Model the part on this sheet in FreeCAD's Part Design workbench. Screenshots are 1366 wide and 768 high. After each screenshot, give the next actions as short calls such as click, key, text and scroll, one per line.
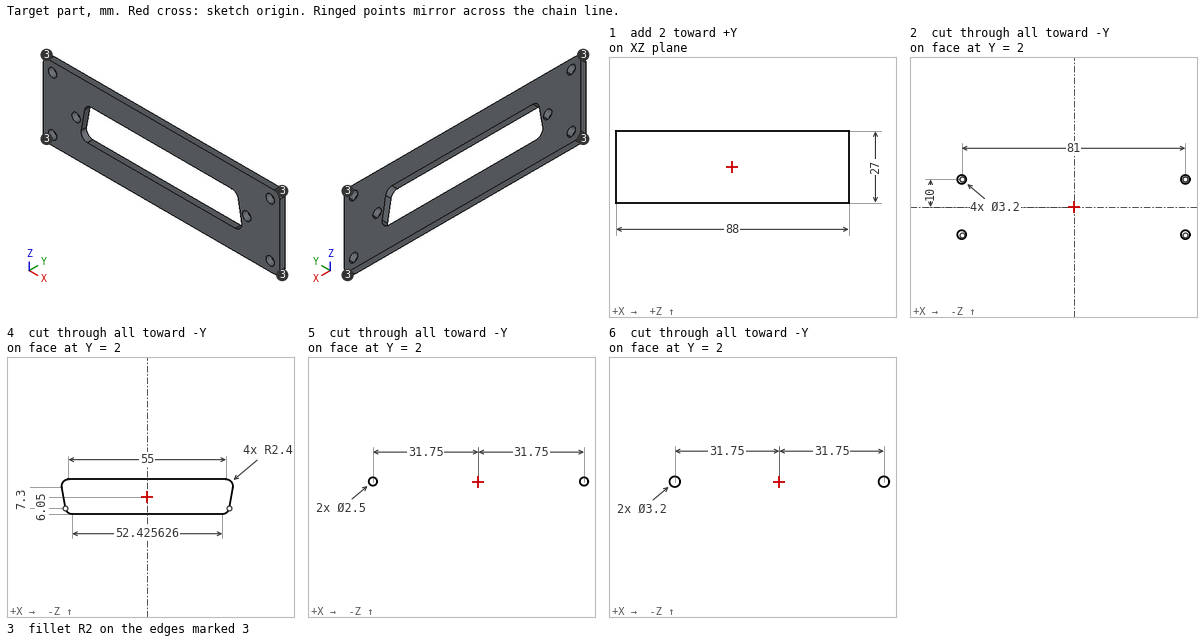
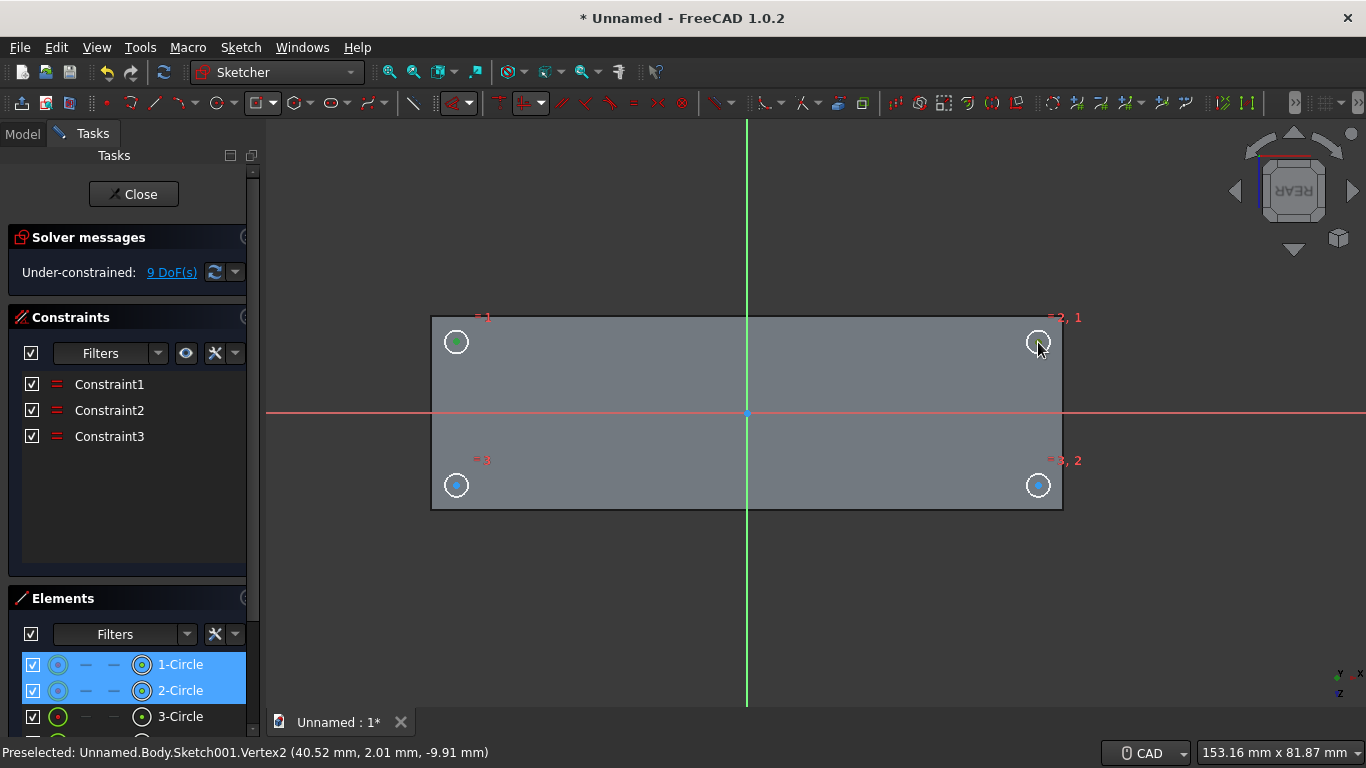
click(747, 641)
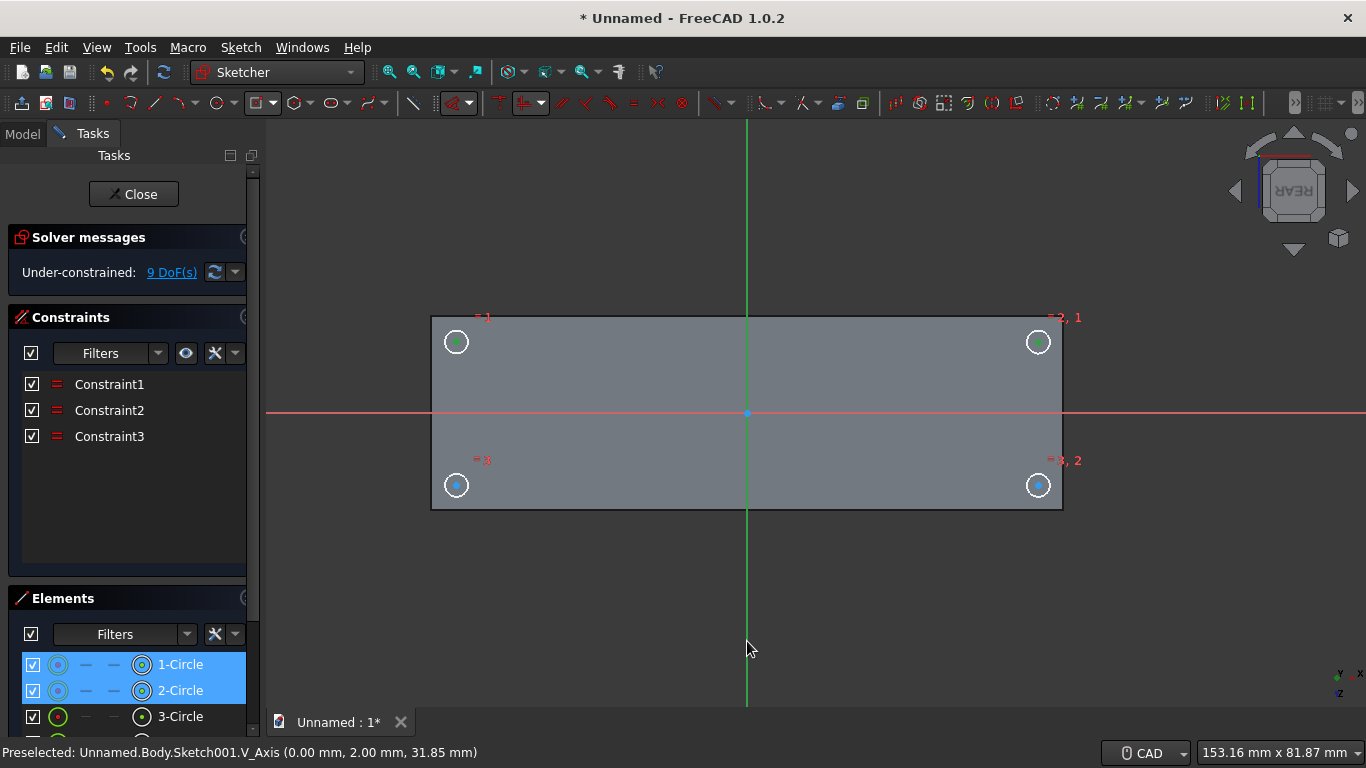
key(s)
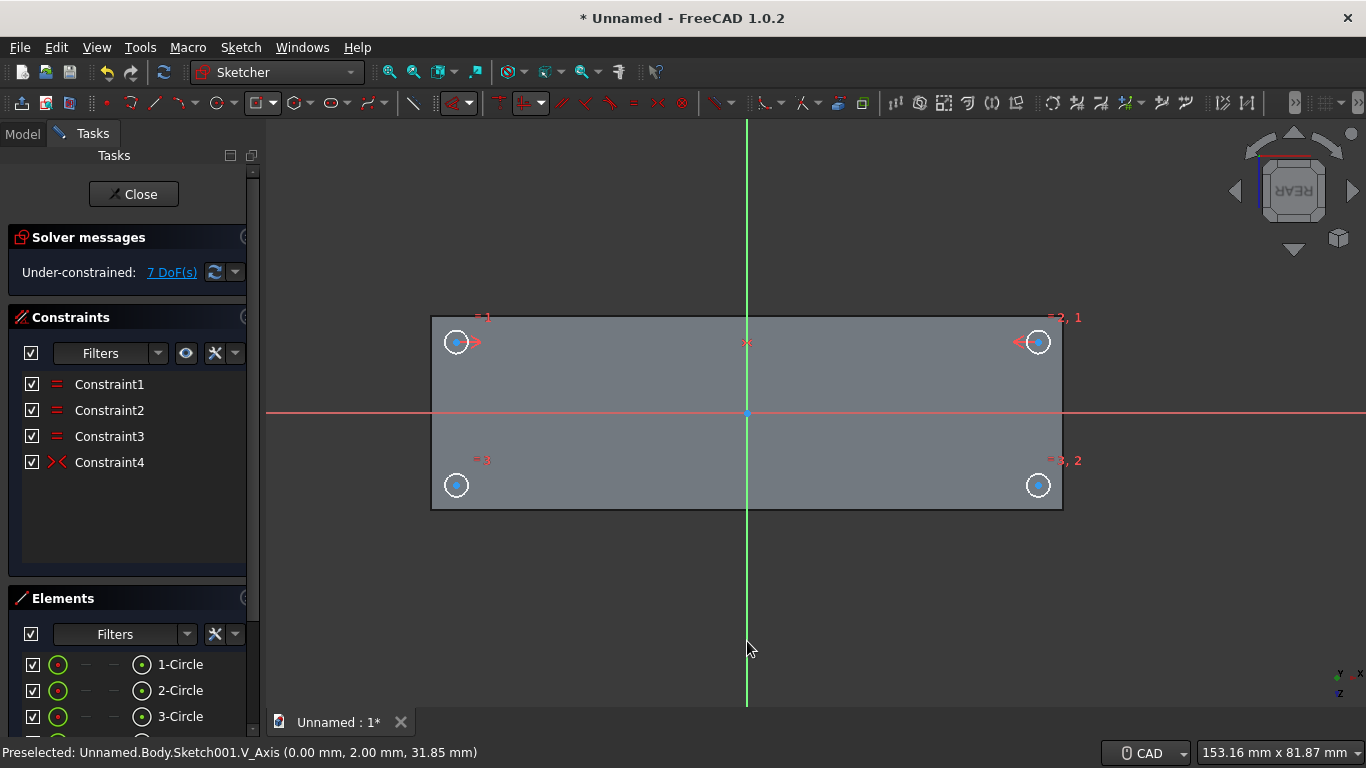
click(1038, 342)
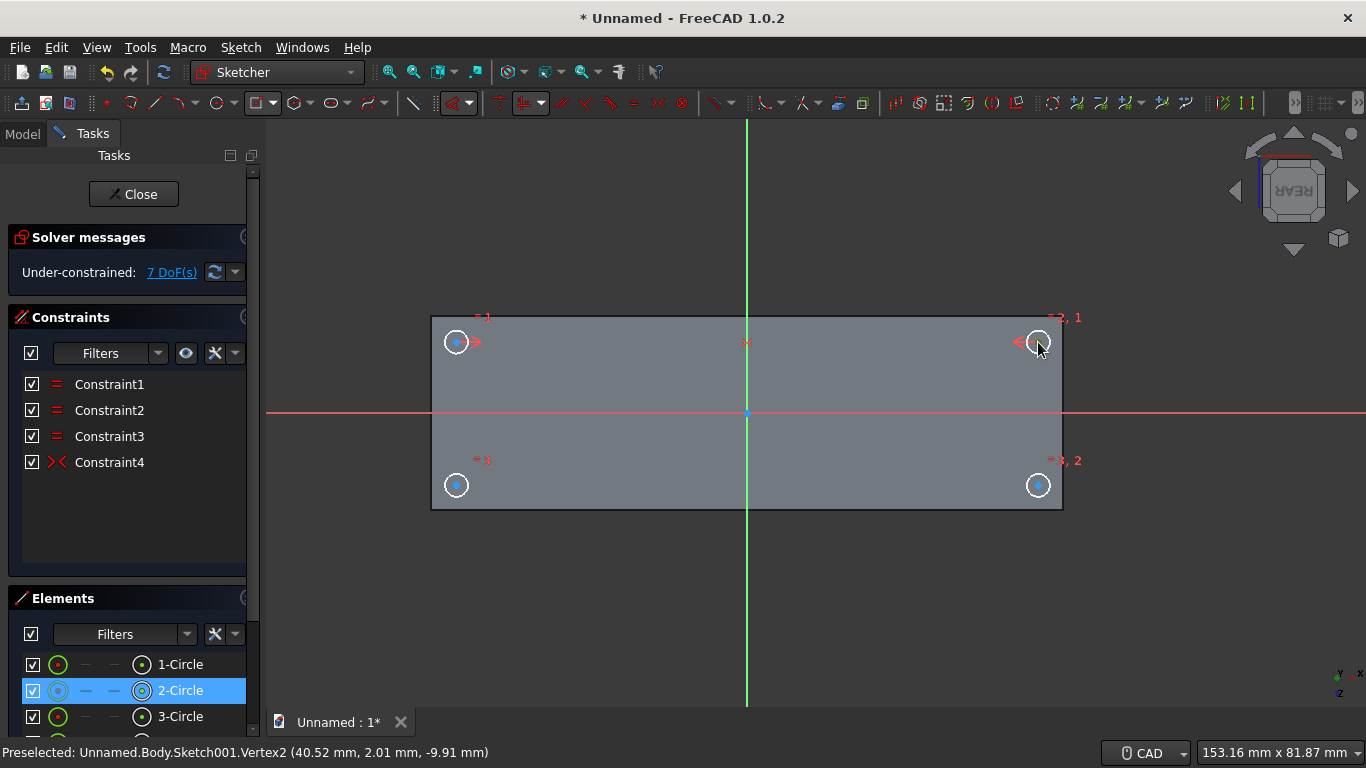
click(1038, 485)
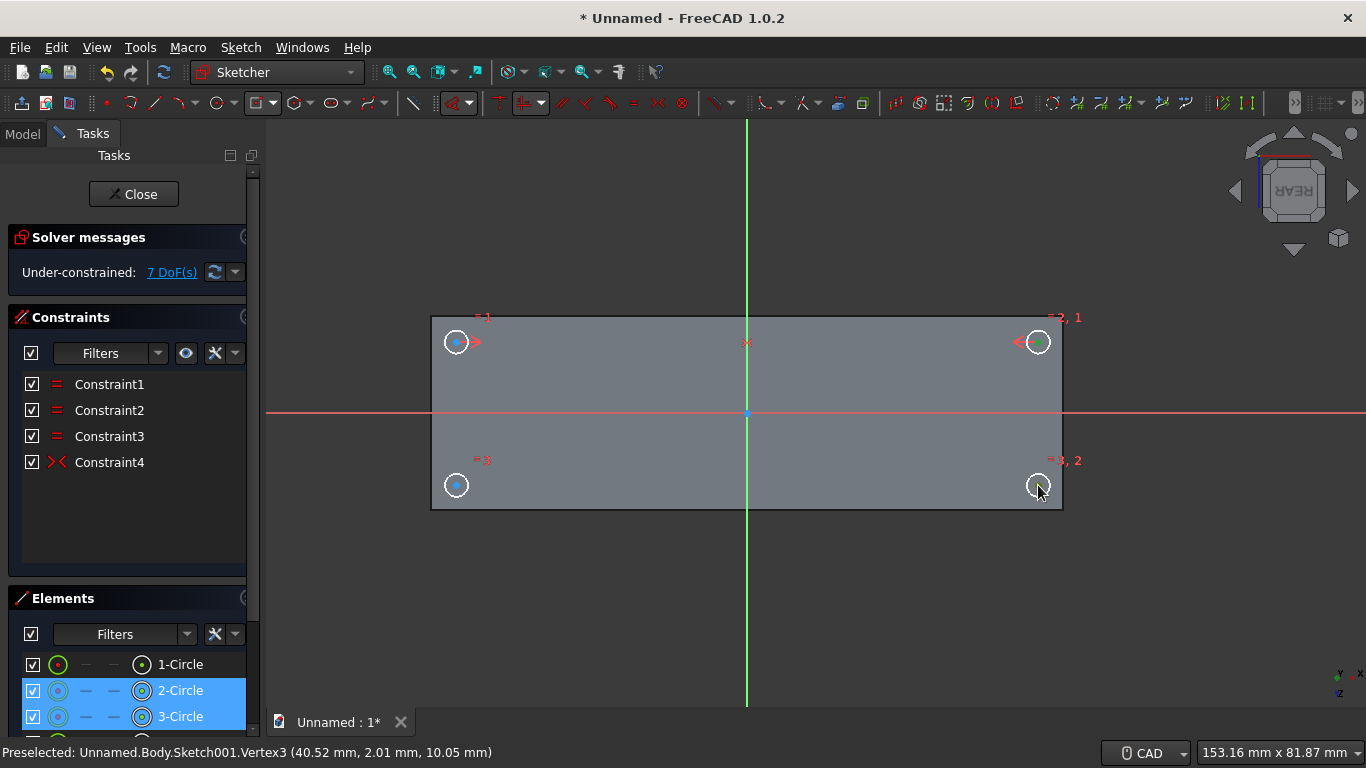
click(359, 413)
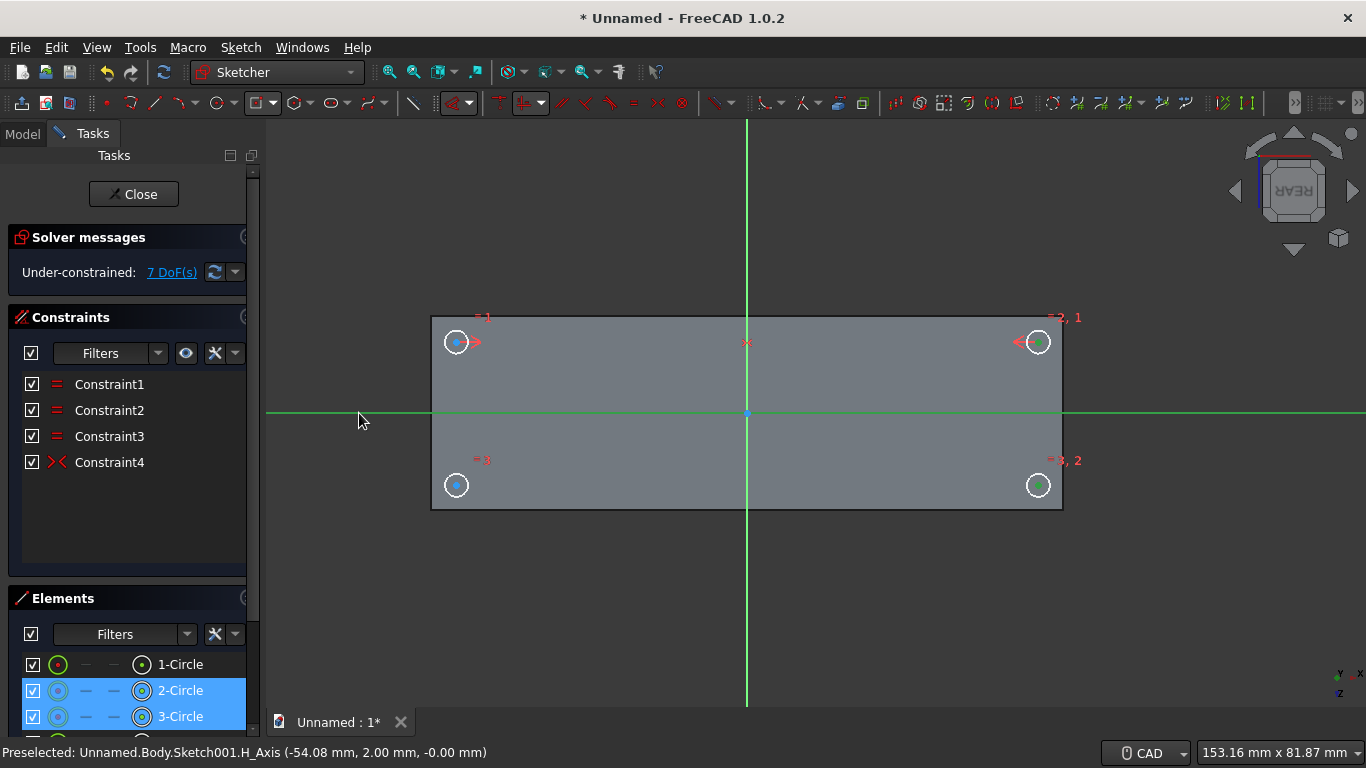
click(658, 104)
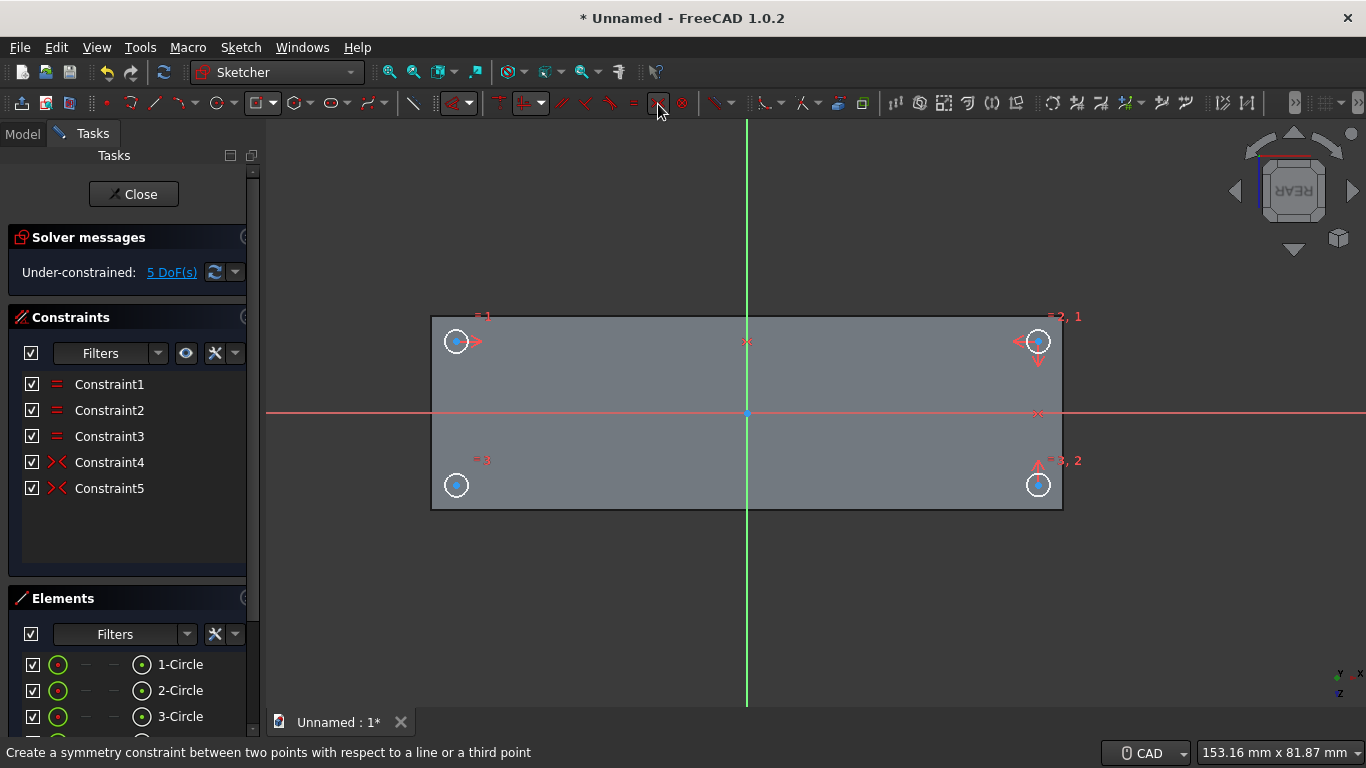
click(456, 342)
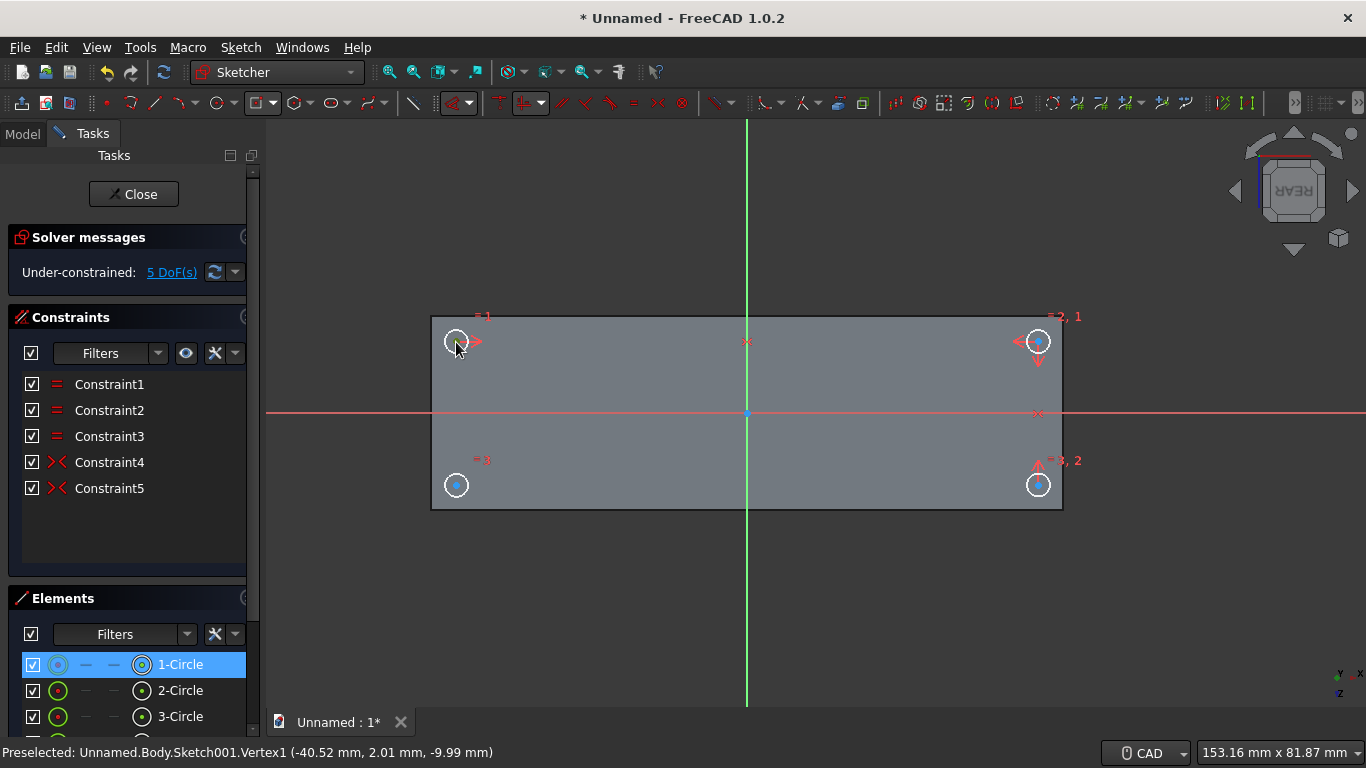
click(457, 485)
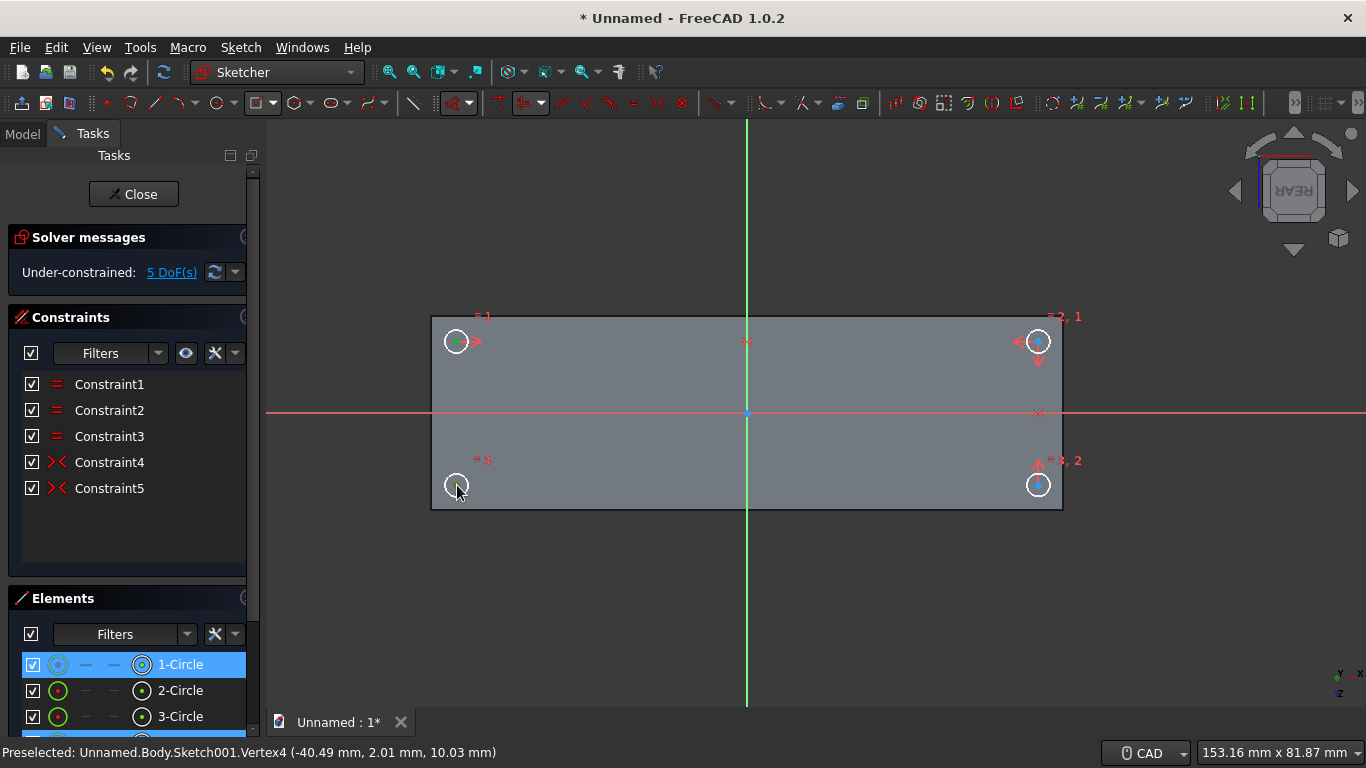
click(359, 413)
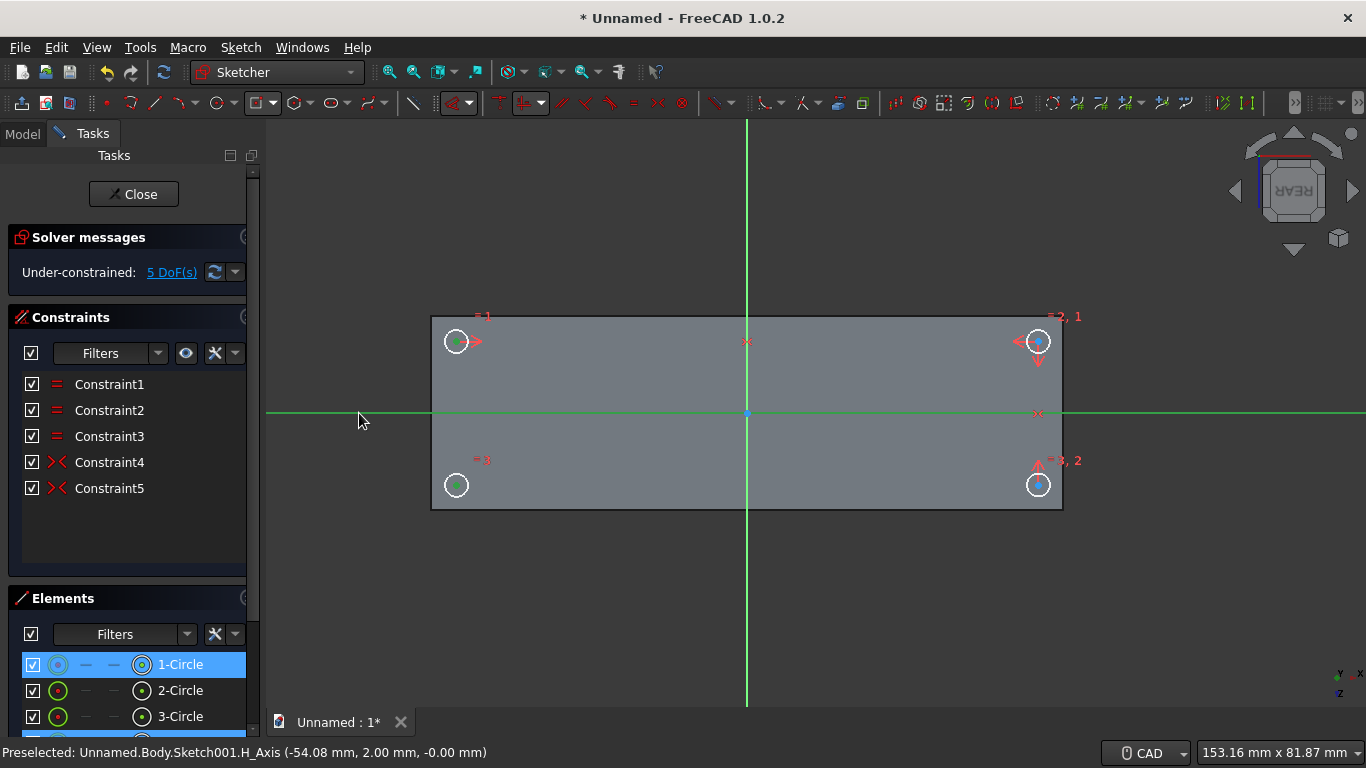
click(658, 104)